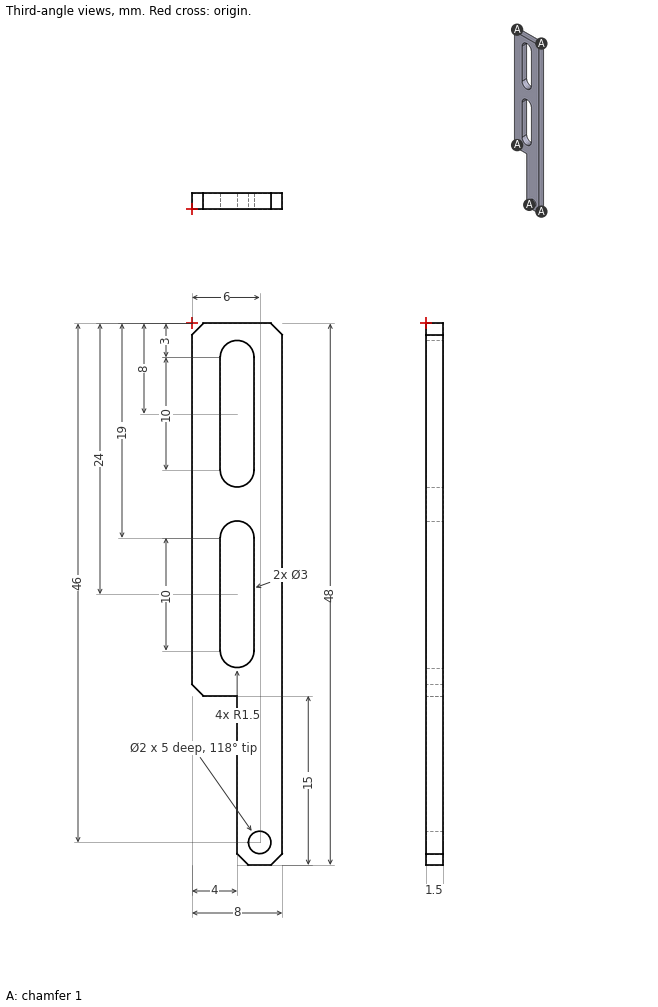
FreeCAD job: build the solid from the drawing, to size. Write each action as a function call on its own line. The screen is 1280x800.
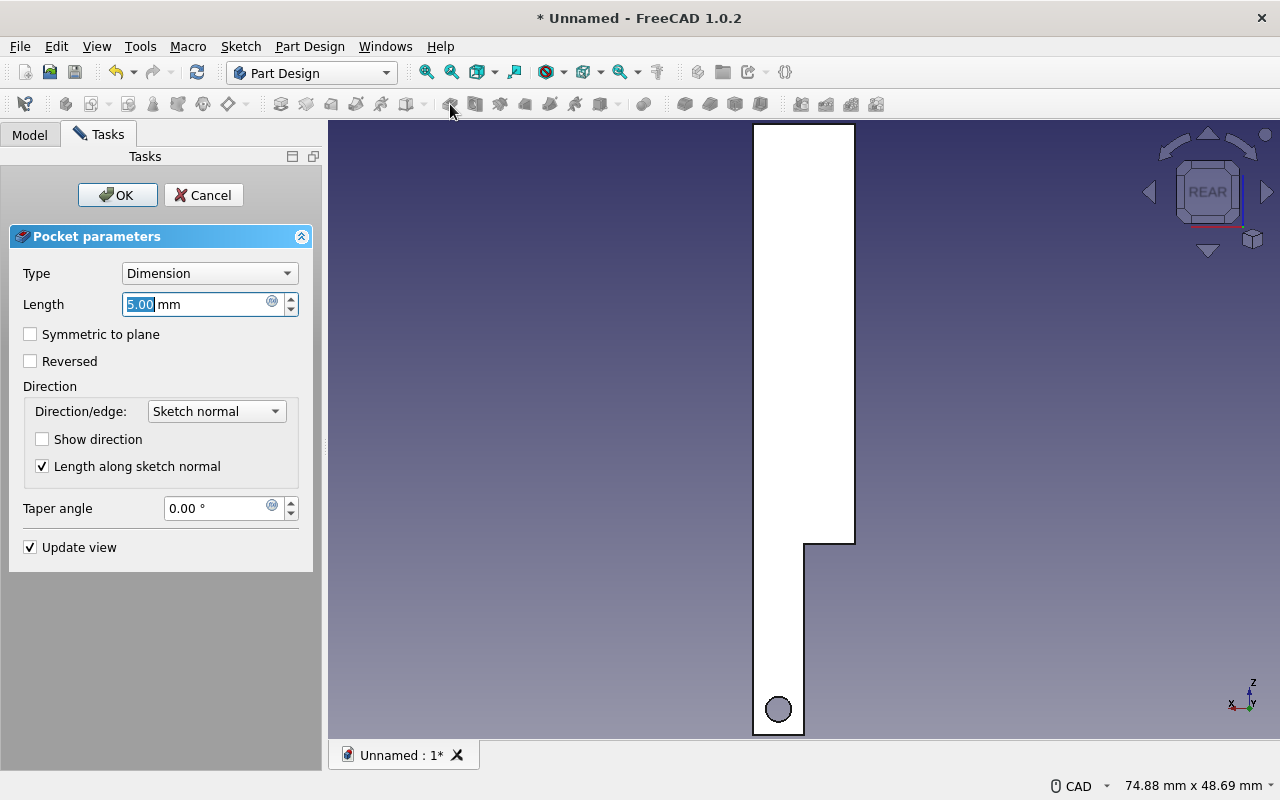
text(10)
key(Tab)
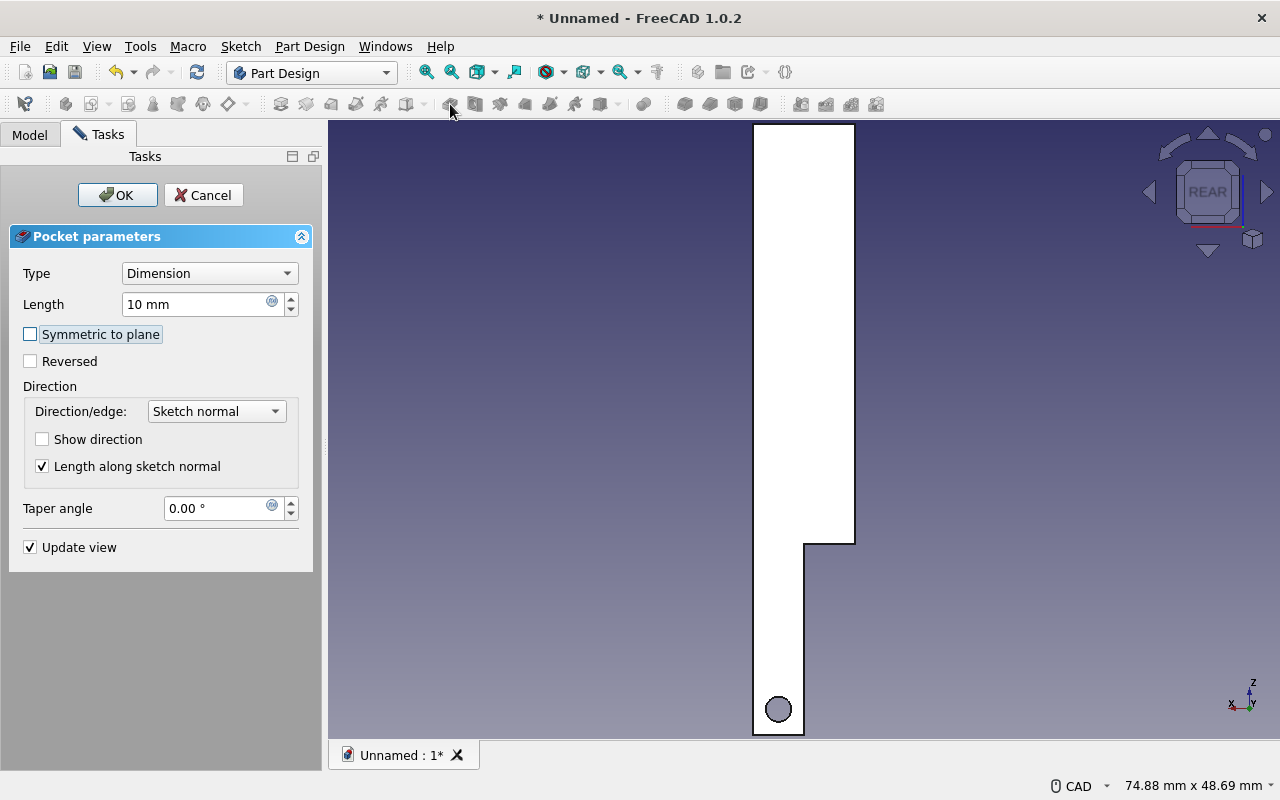
click(118, 195)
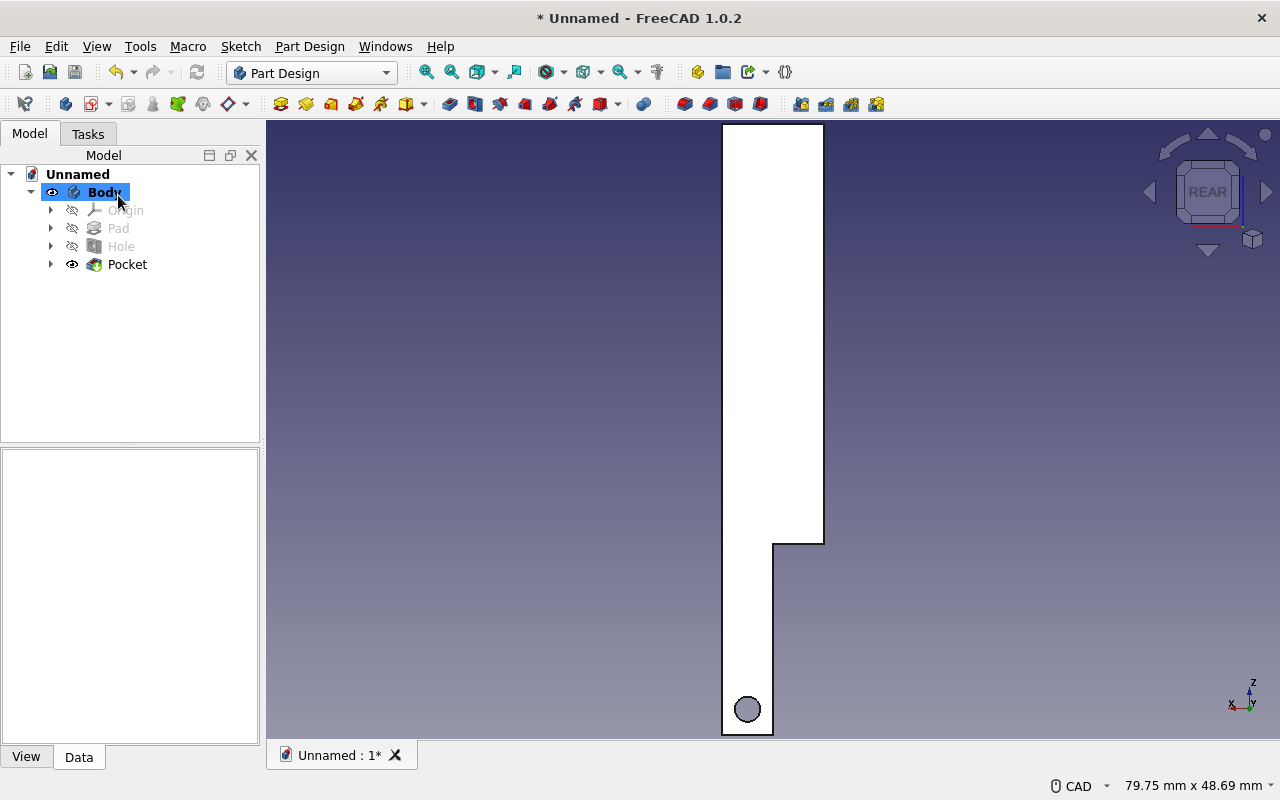
click(773, 254)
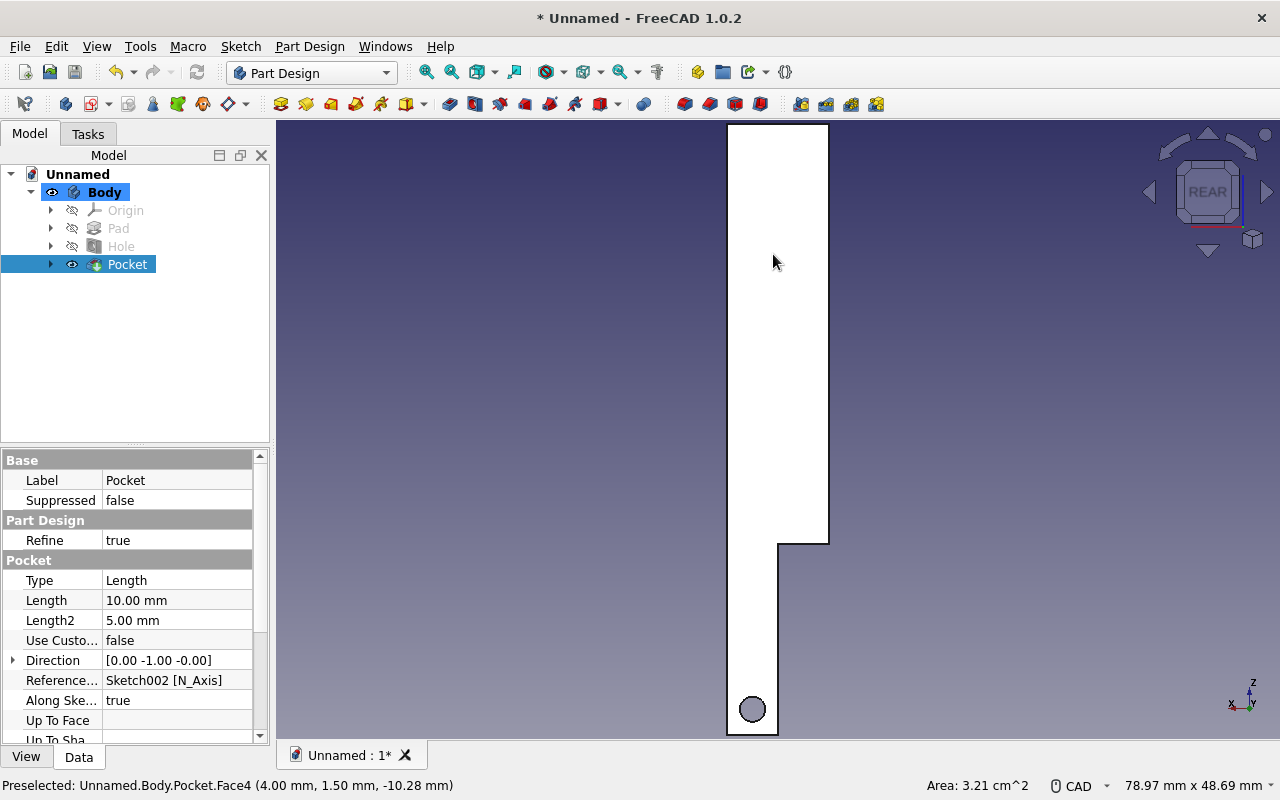
click(90, 104)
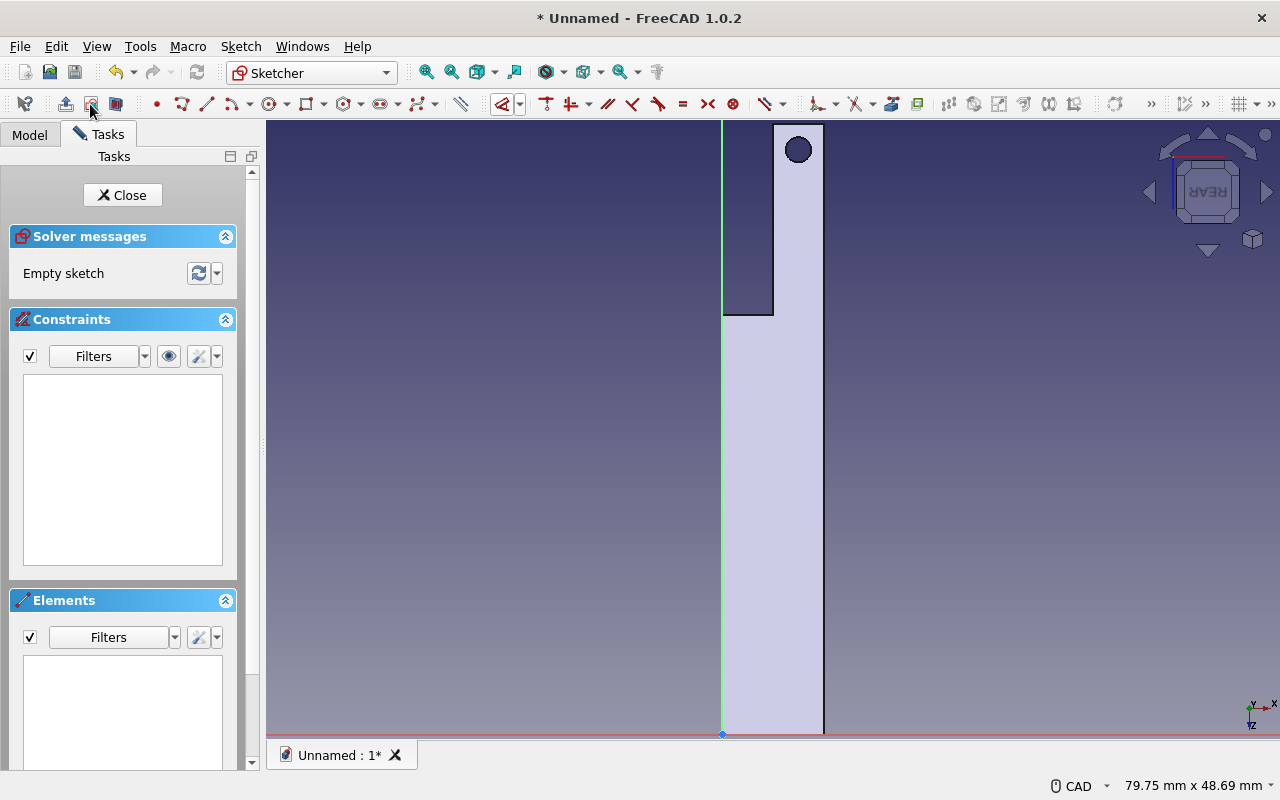
scroll(467, 148, down, 1)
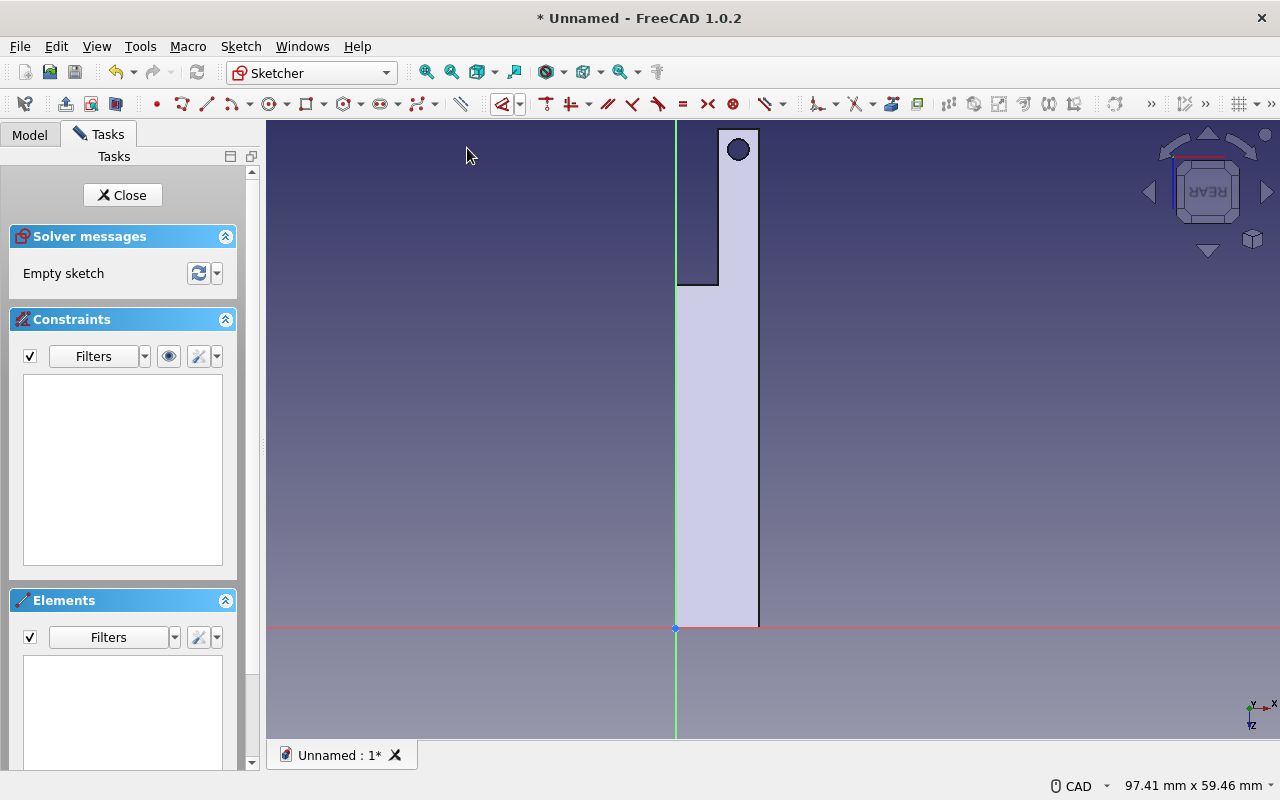
scroll(705, 630, up, 2)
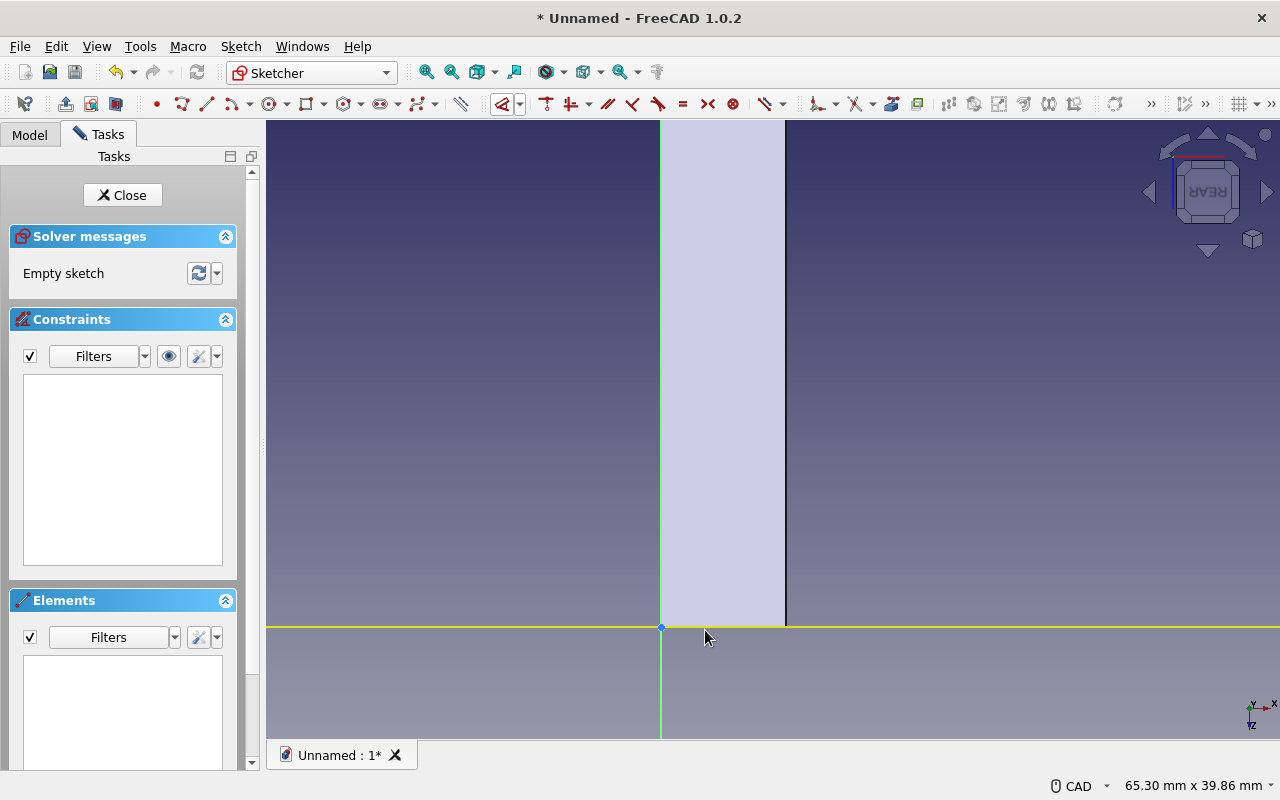
click(268, 104)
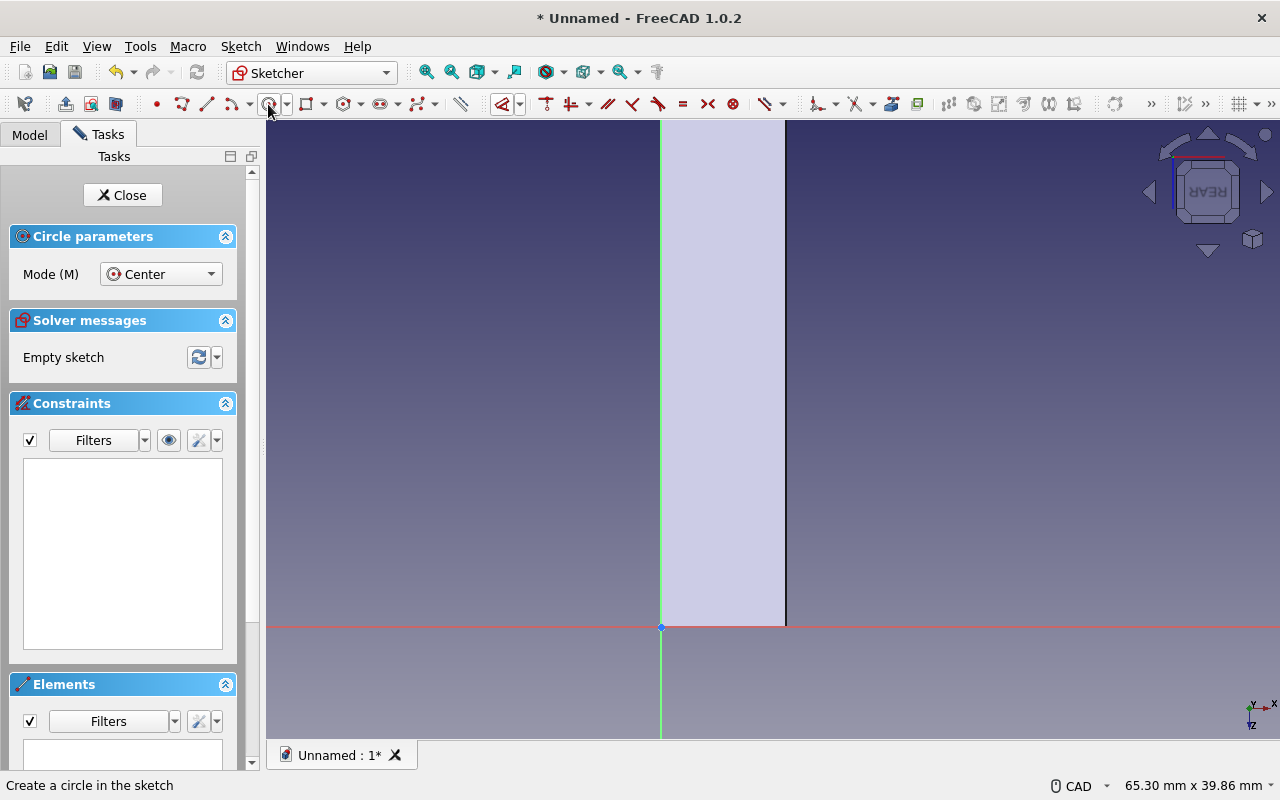
click(724, 254)
move(740, 238)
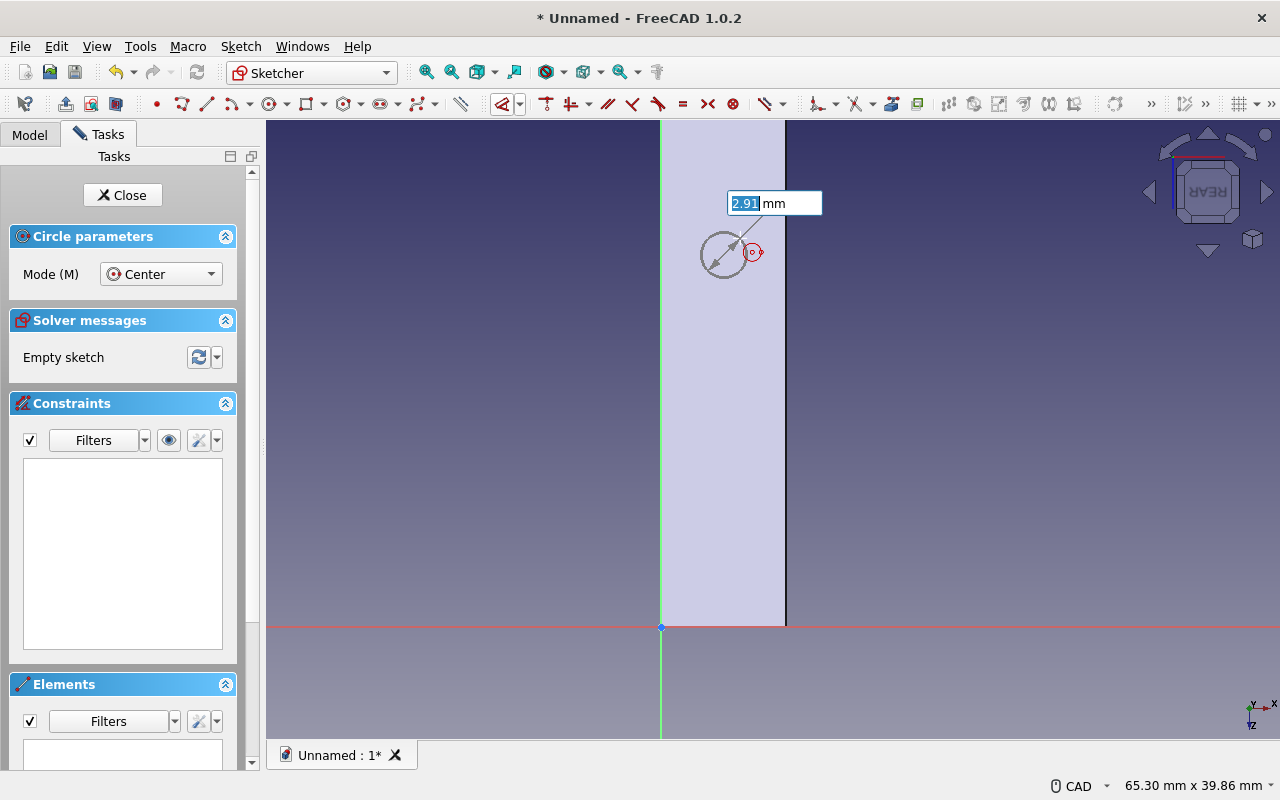
text(3)
key(Return)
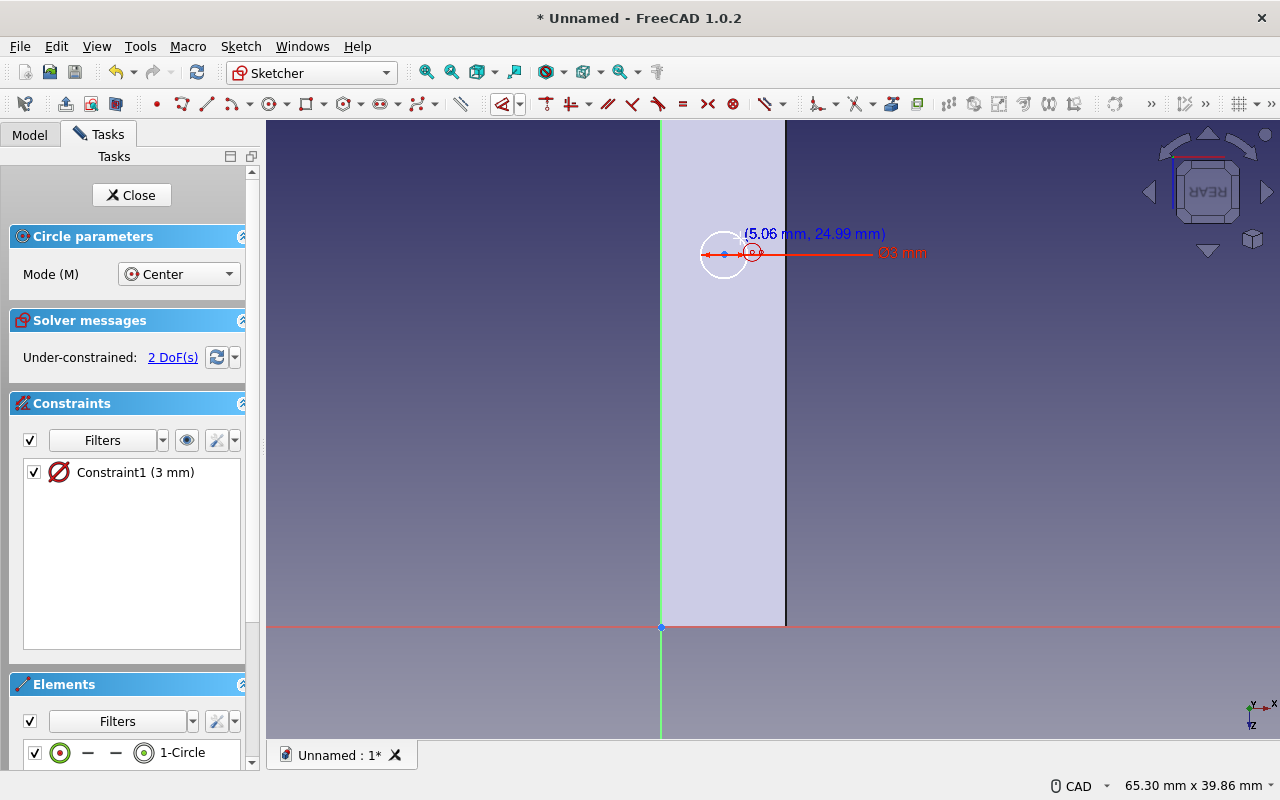
click(724, 503)
move(740, 486)